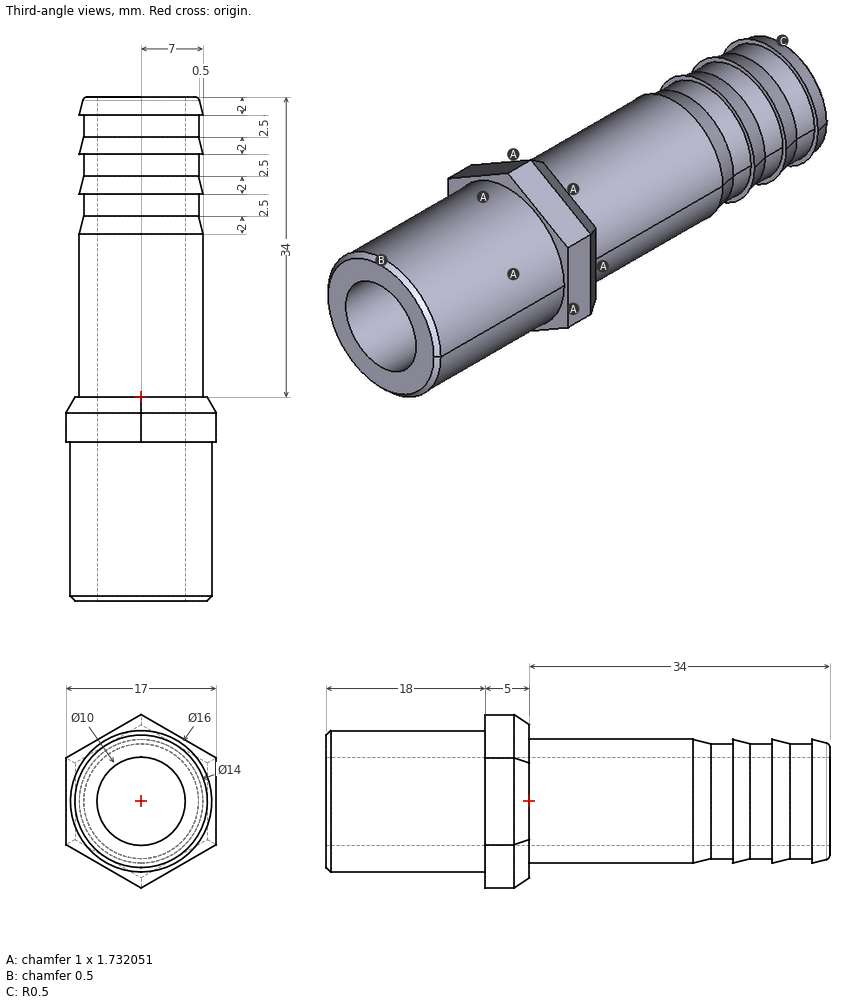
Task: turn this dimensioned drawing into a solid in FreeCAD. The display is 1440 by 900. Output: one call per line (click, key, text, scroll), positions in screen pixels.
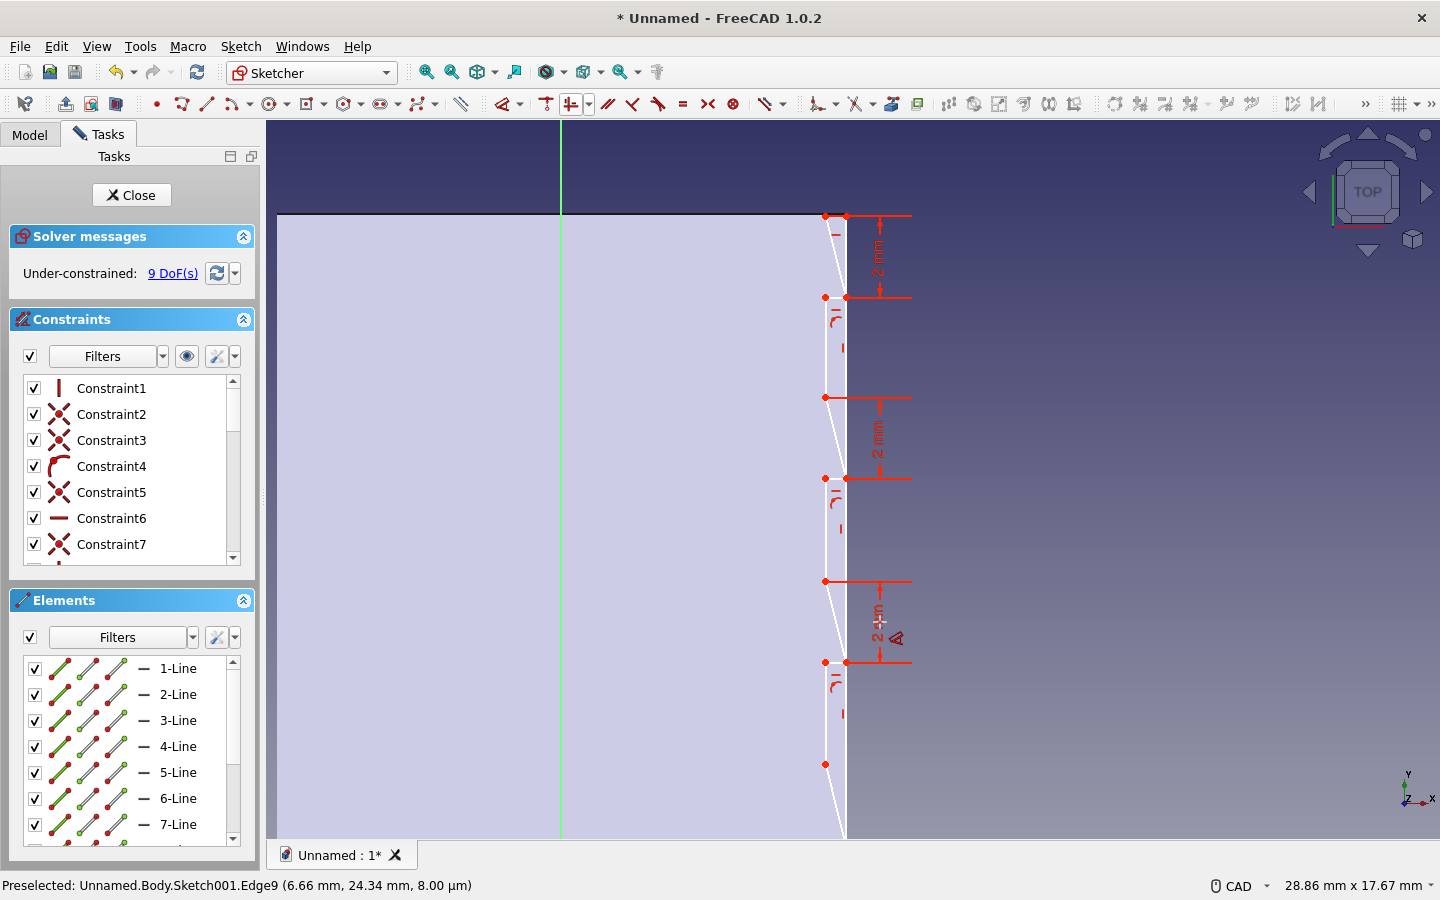
click(832, 789)
click(880, 788)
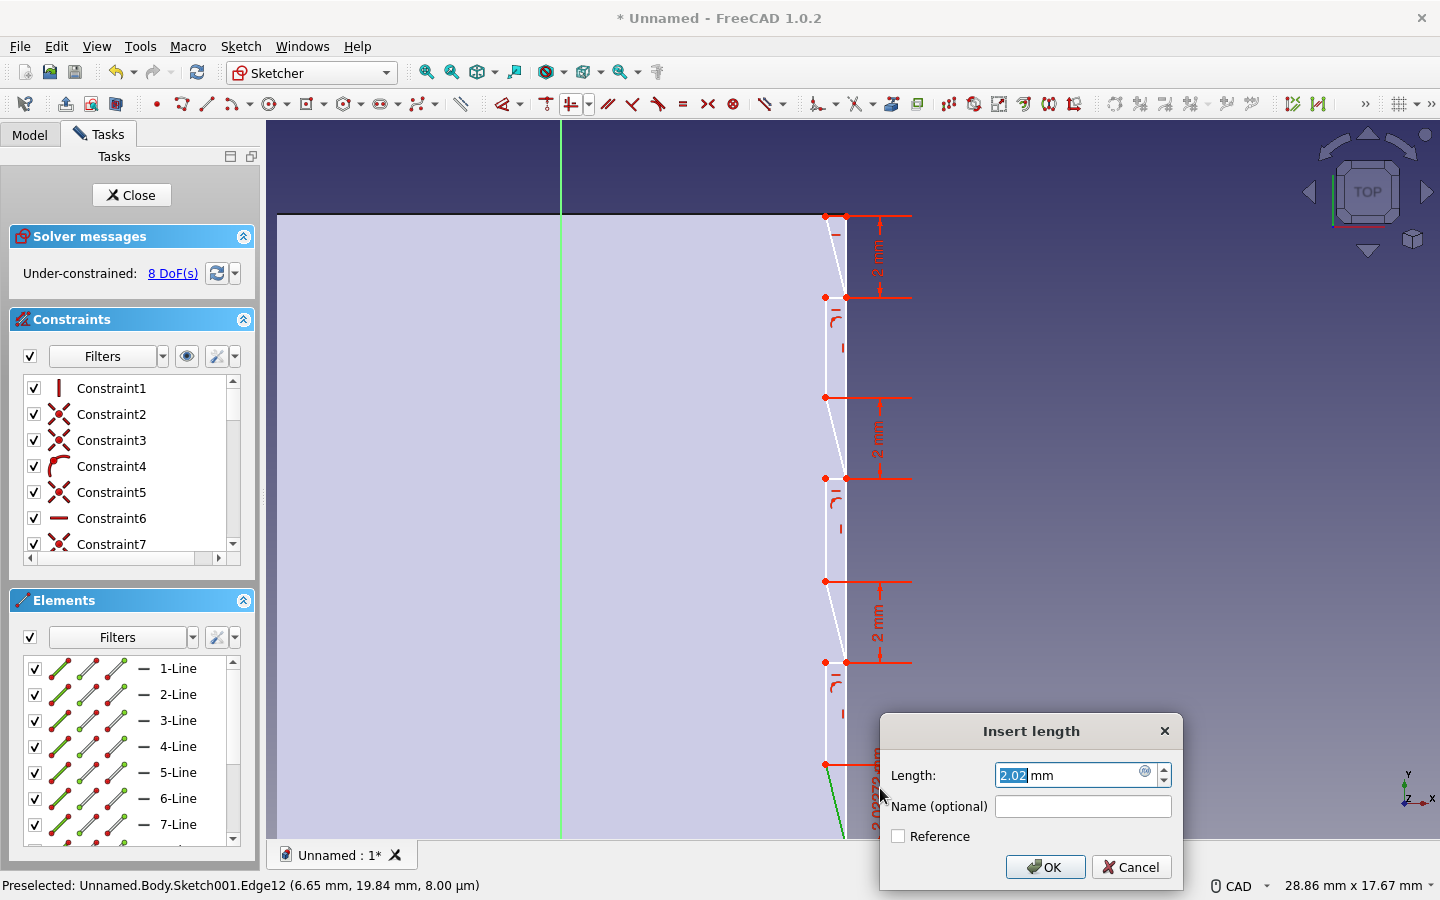
text(2)
key(Return)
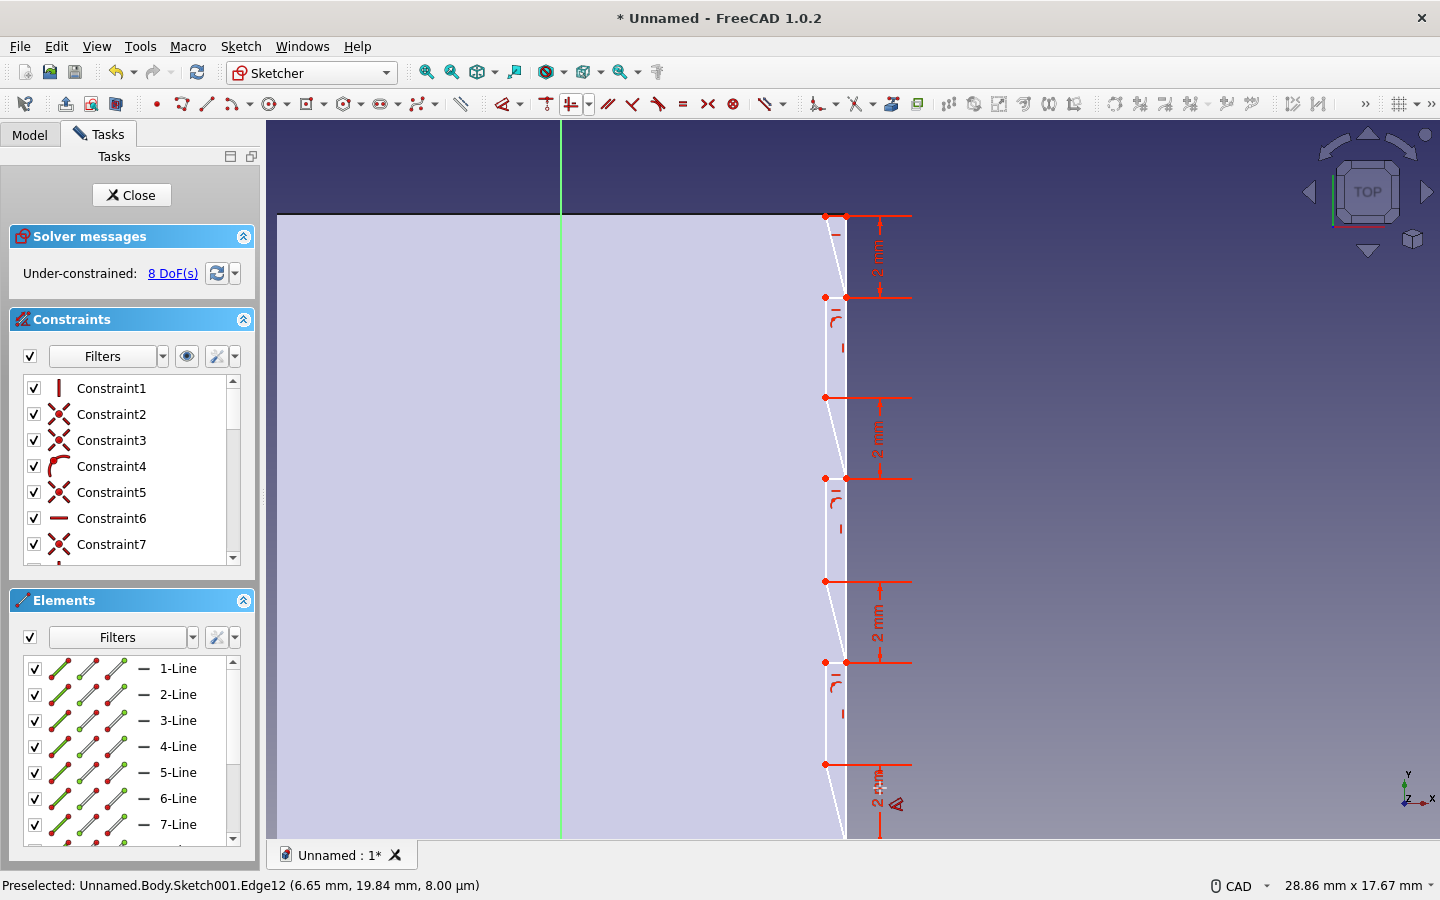
scroll(836, 216, up, 4)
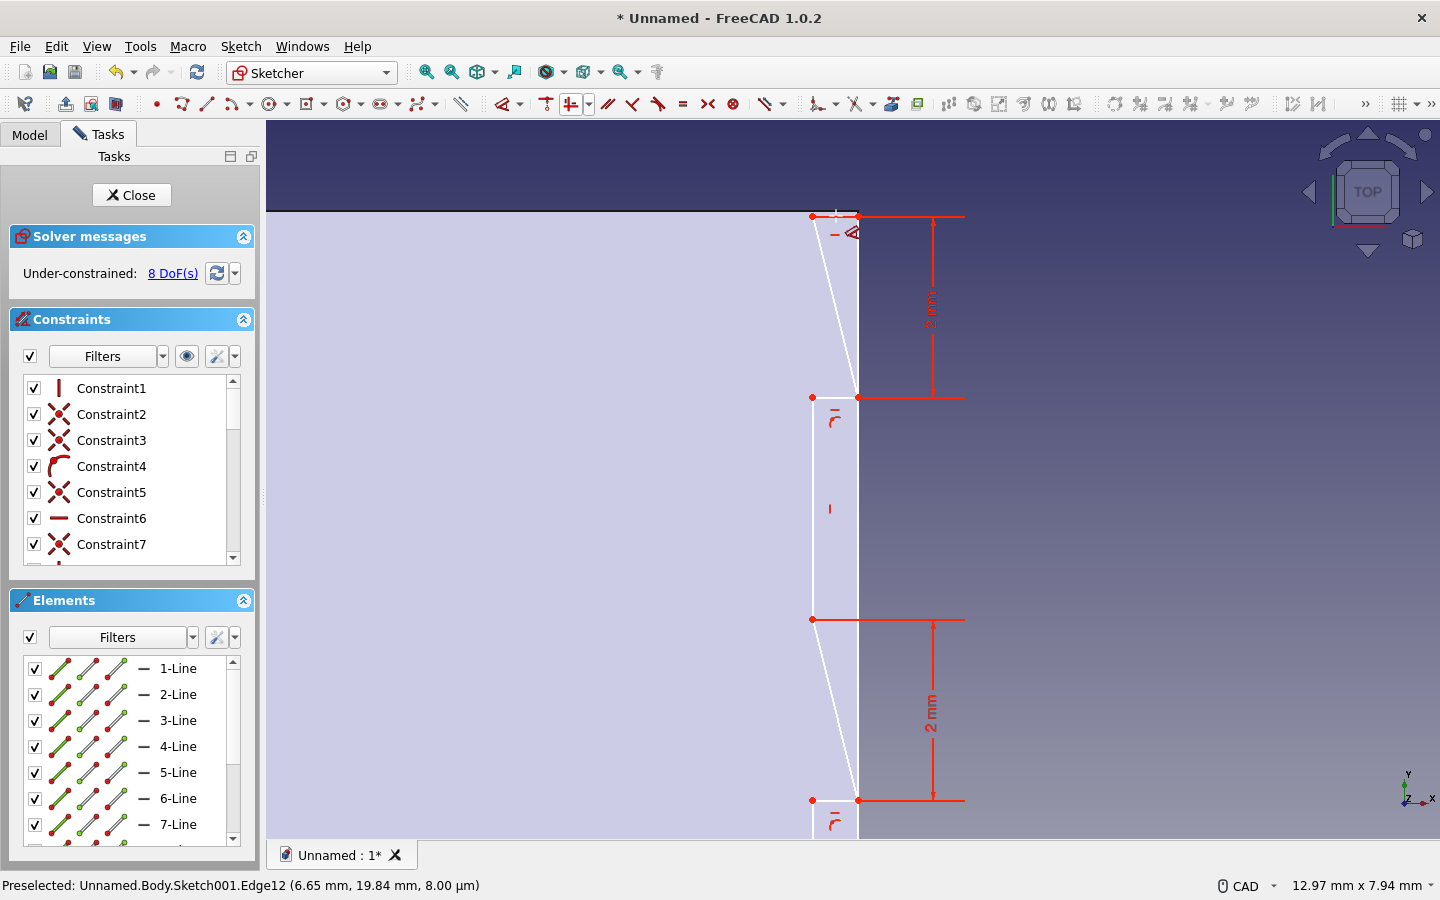
click(835, 217)
click(835, 183)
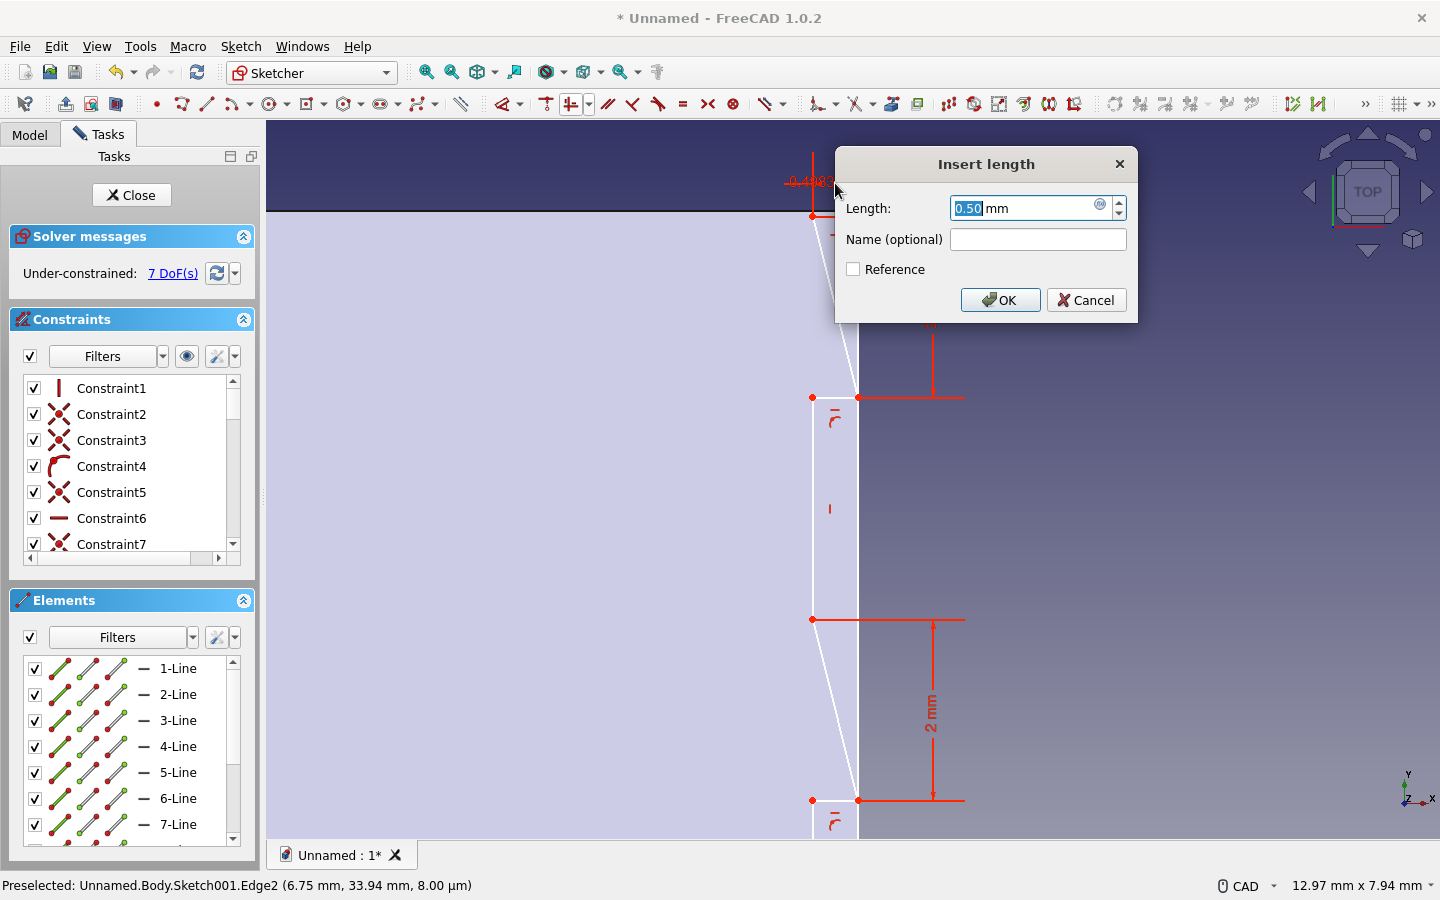
text(0.5)
key(Return)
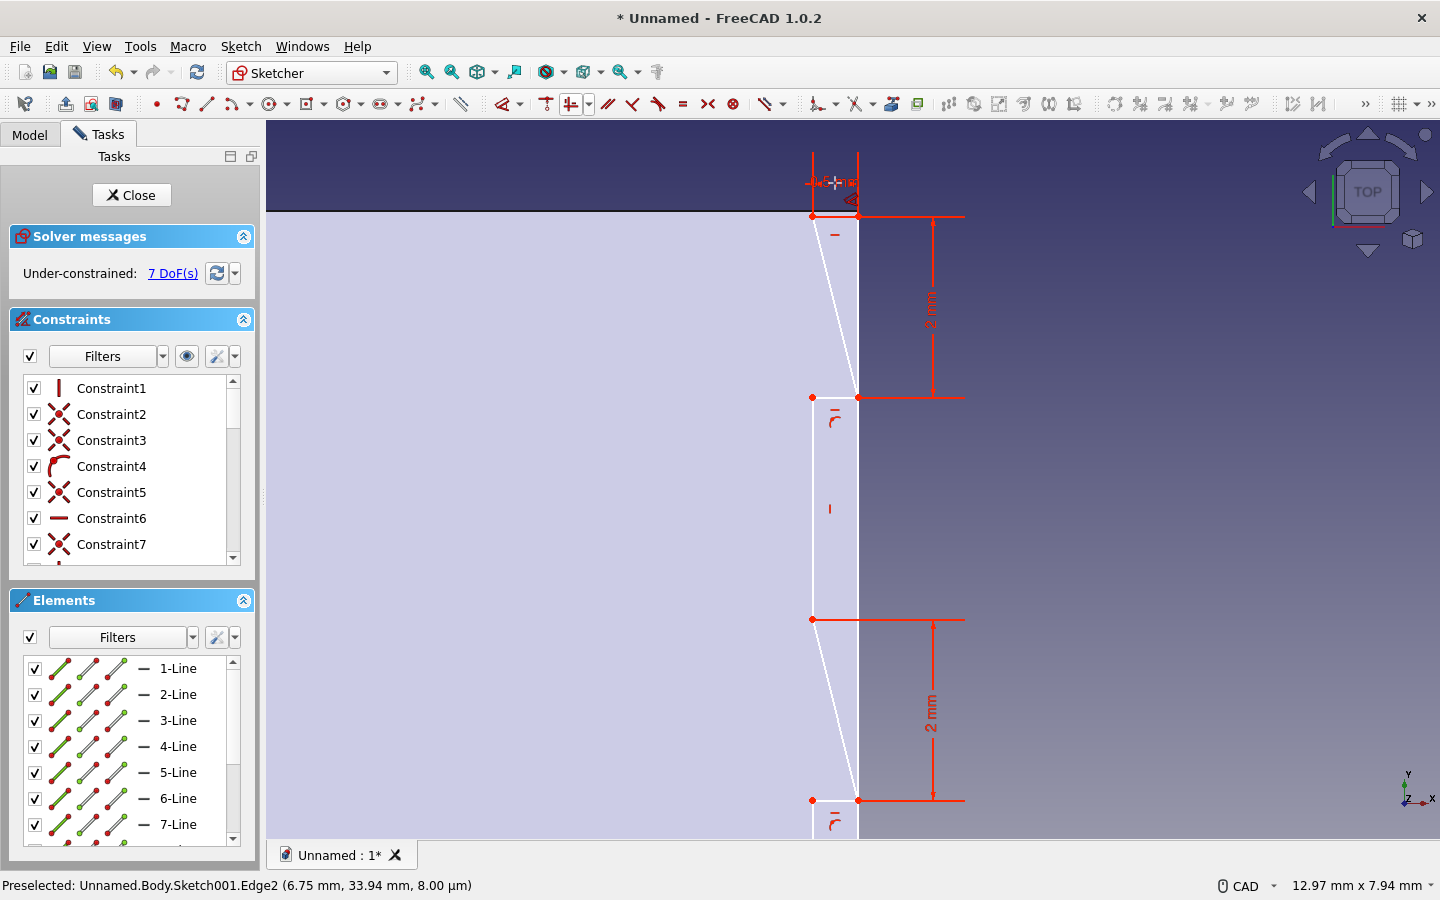
click(845, 398)
click(835, 364)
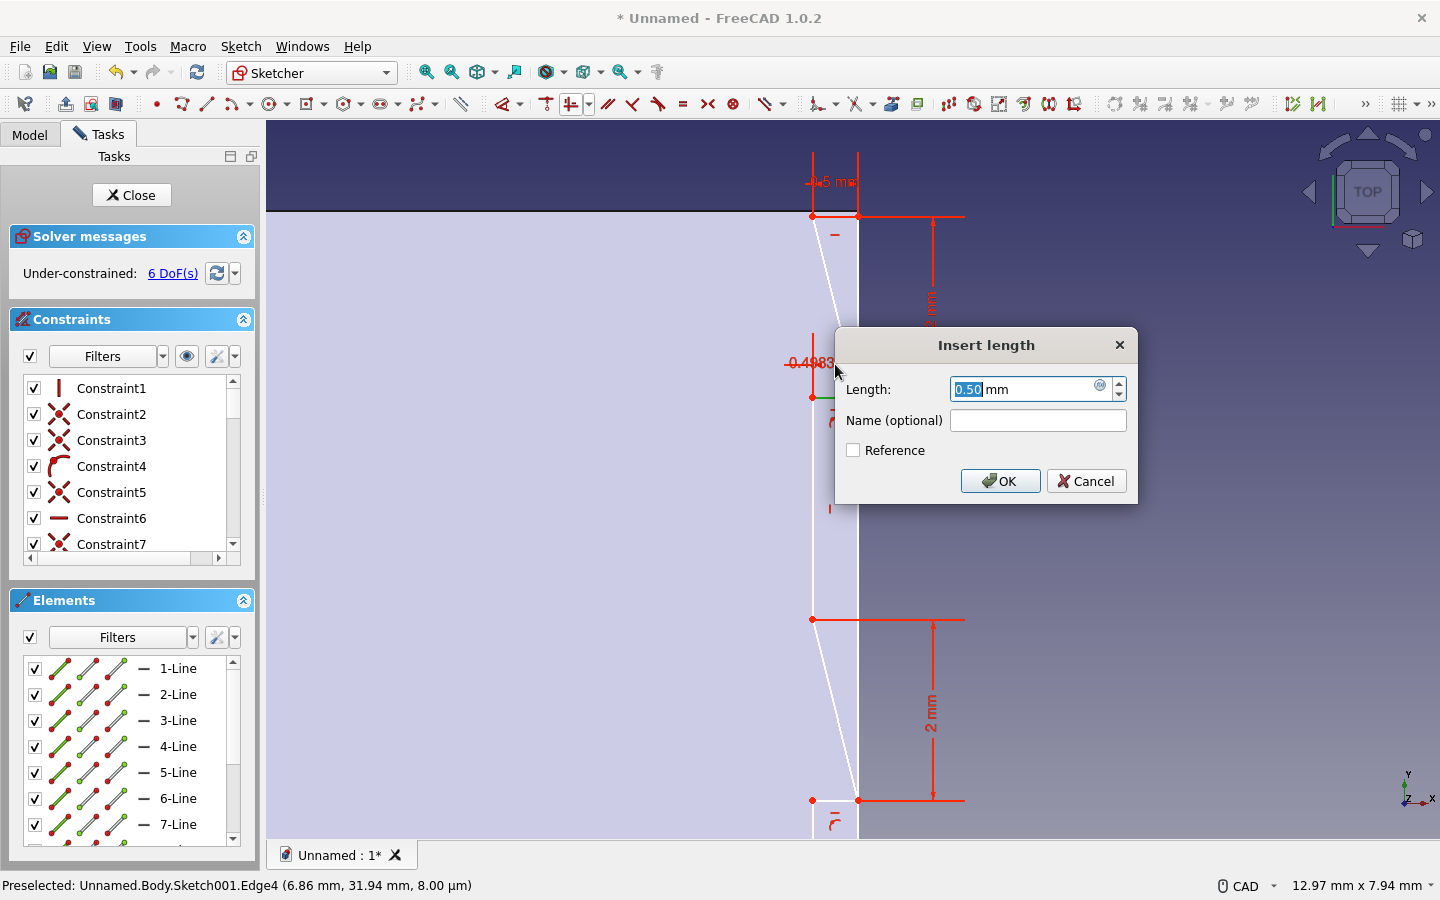
text(0.5)
key(Return)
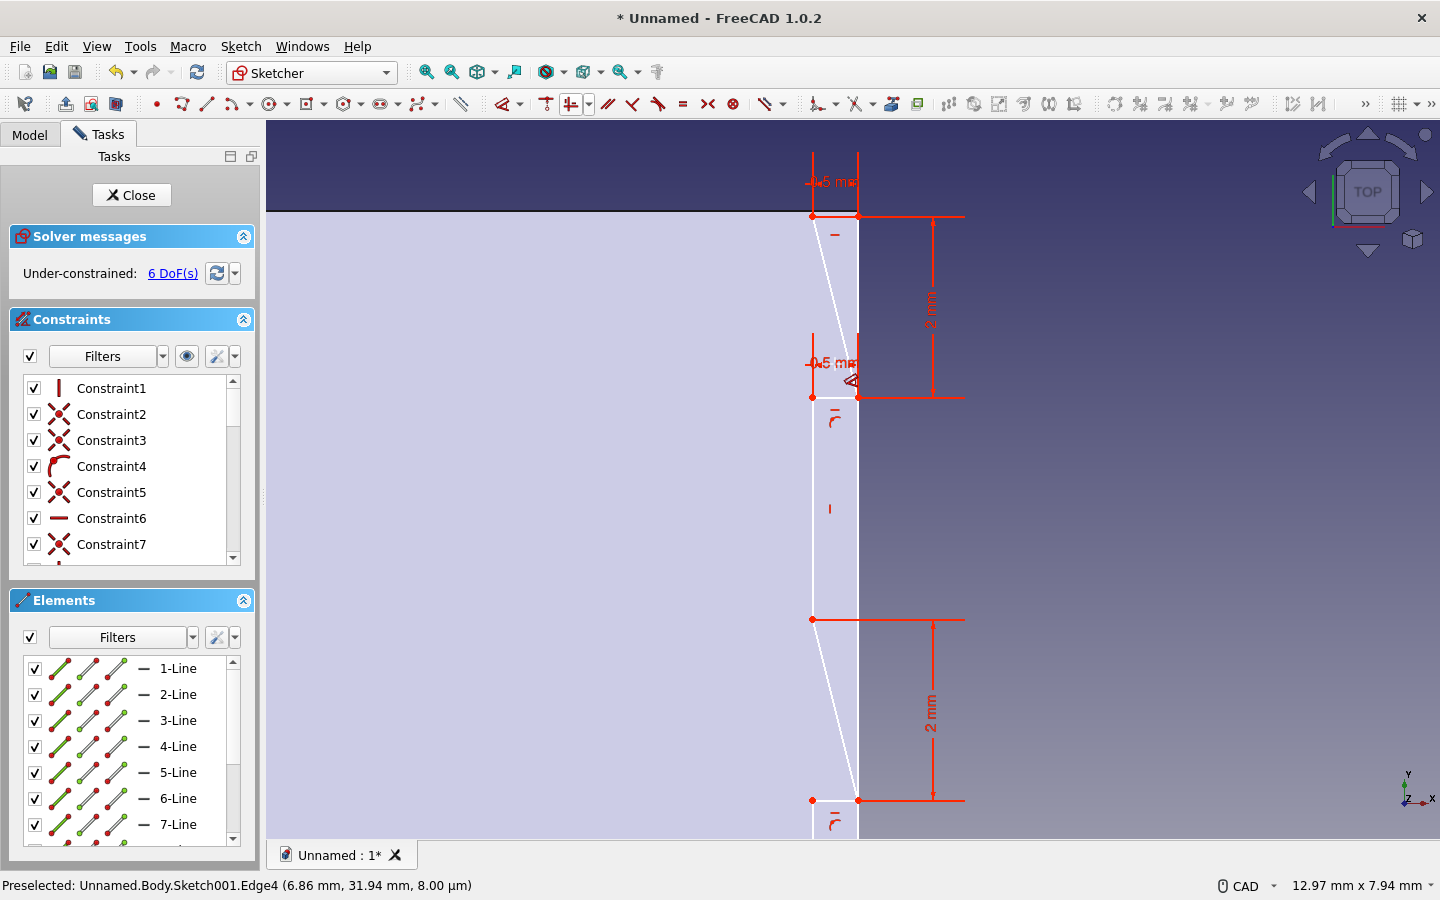
scroll(833, 228, down, 9)